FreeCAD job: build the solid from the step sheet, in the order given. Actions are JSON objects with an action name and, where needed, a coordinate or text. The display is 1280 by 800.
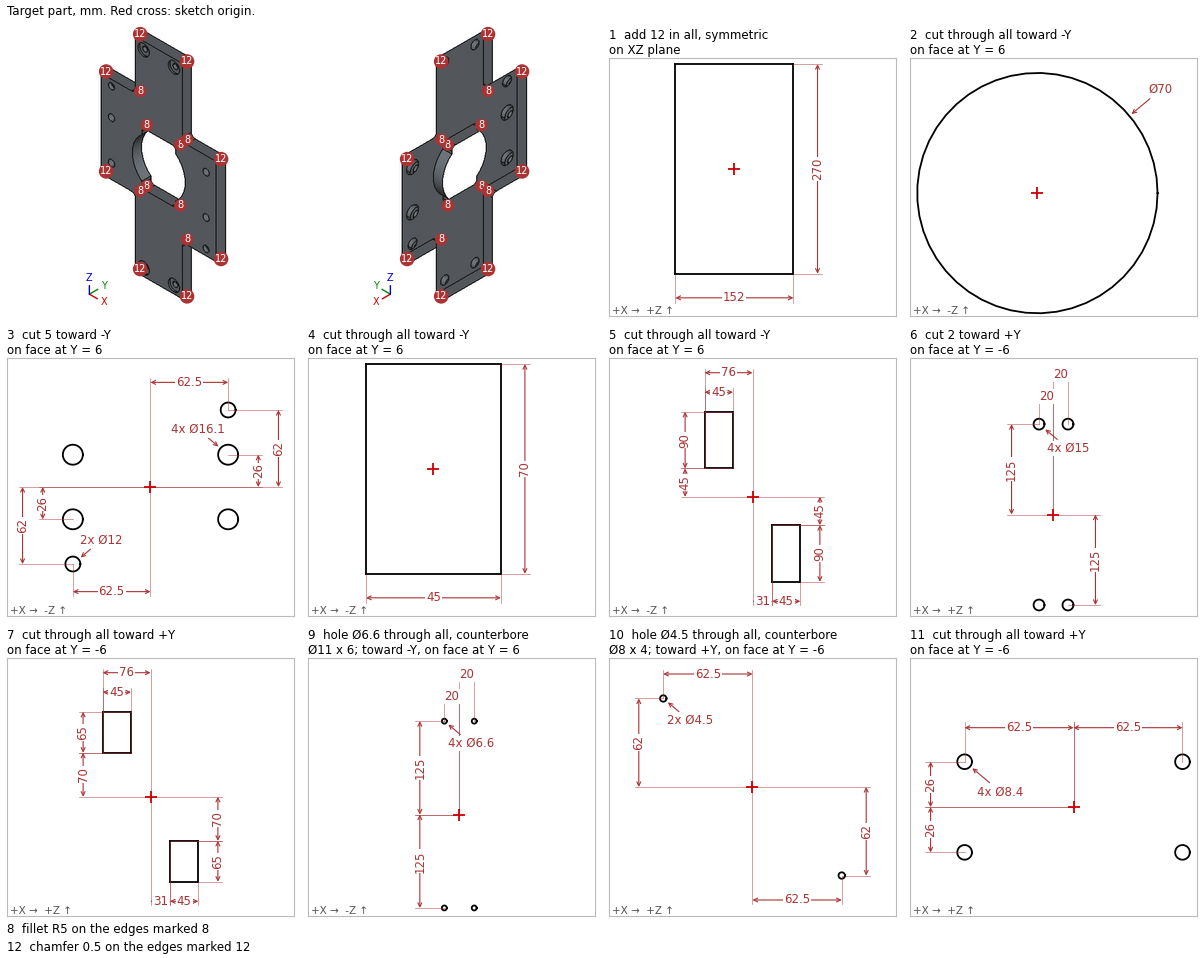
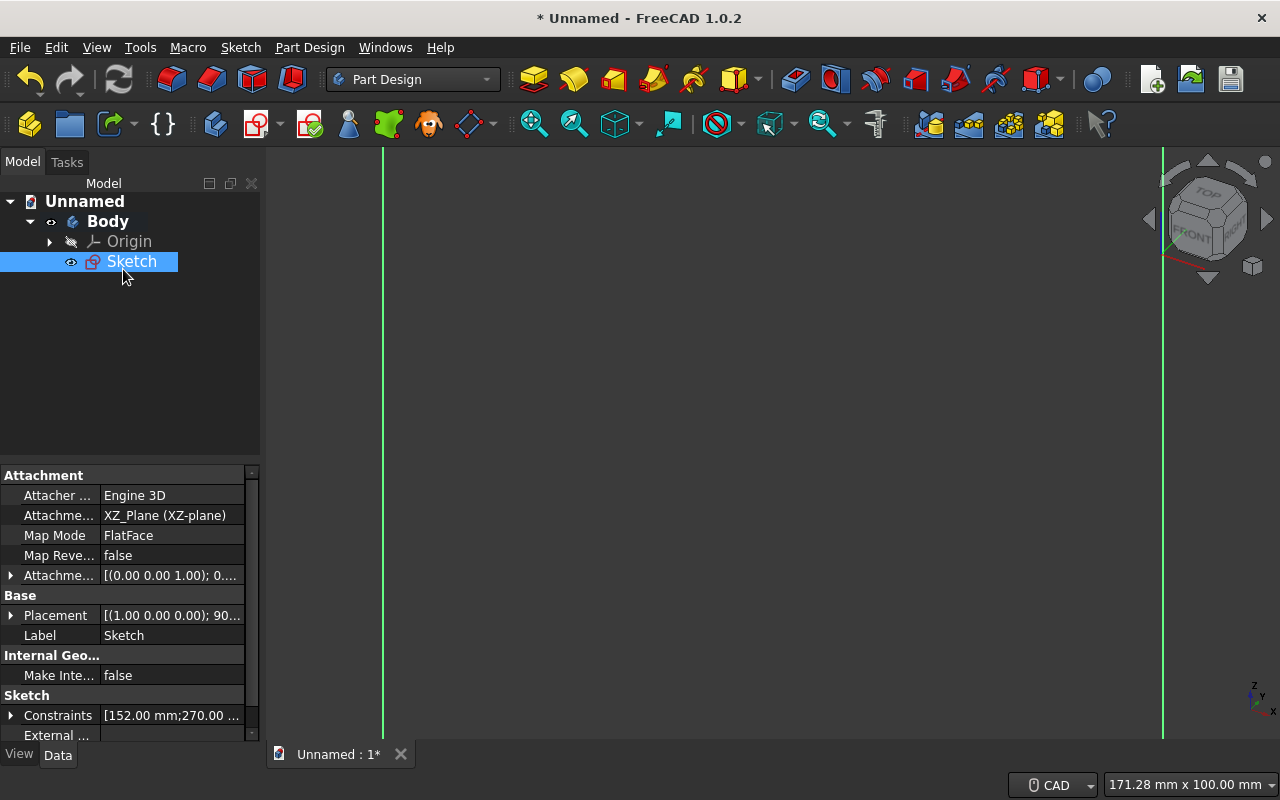
{"action": "left_click", "coordinate": [534, 80]}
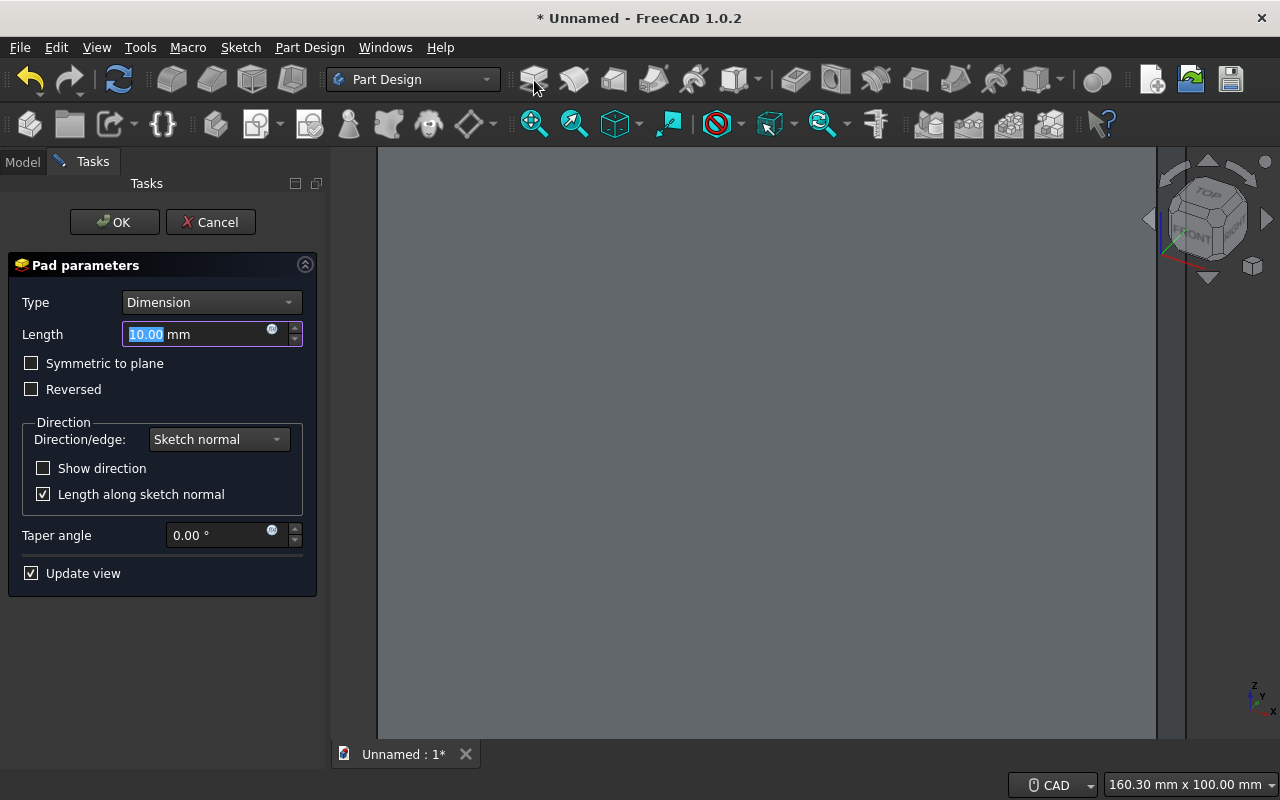
{"action": "type", "text": "12"}
{"action": "key", "text": "Tab"}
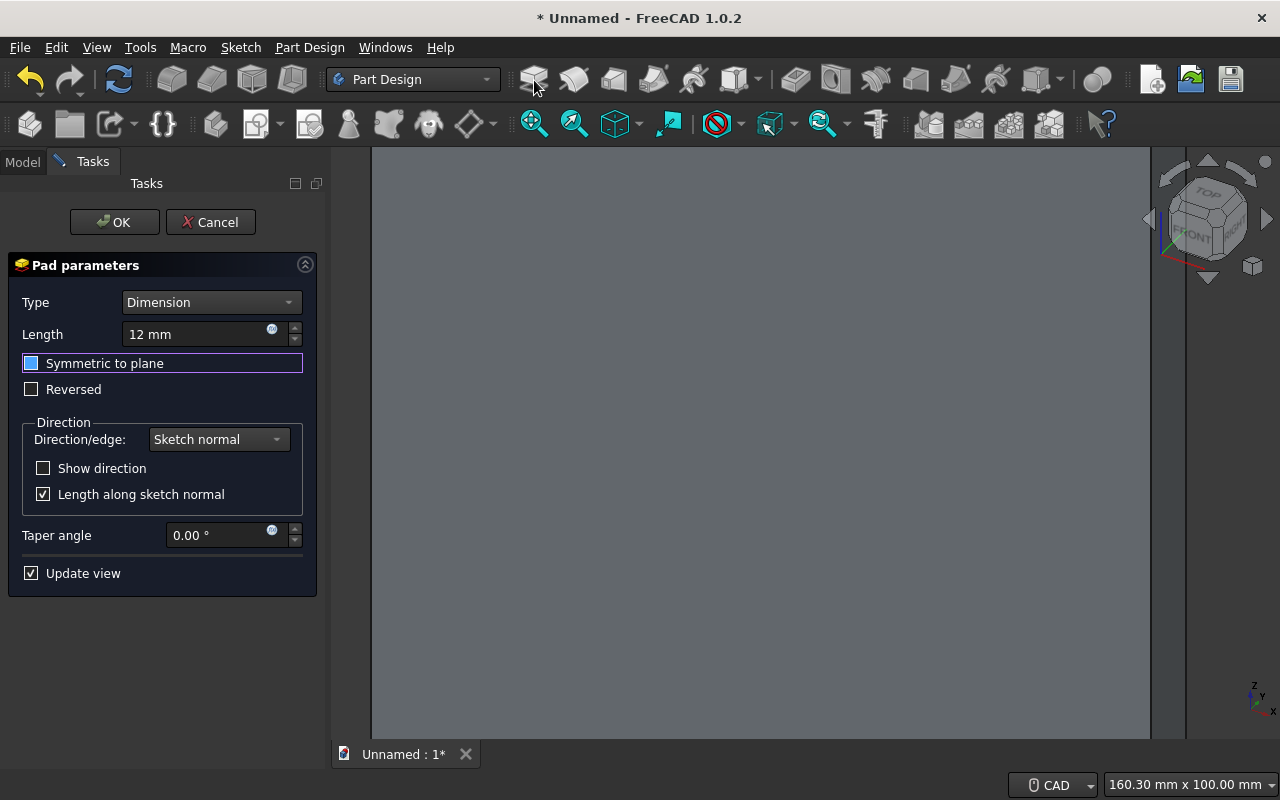
{"action": "left_click", "coordinate": [30, 363]}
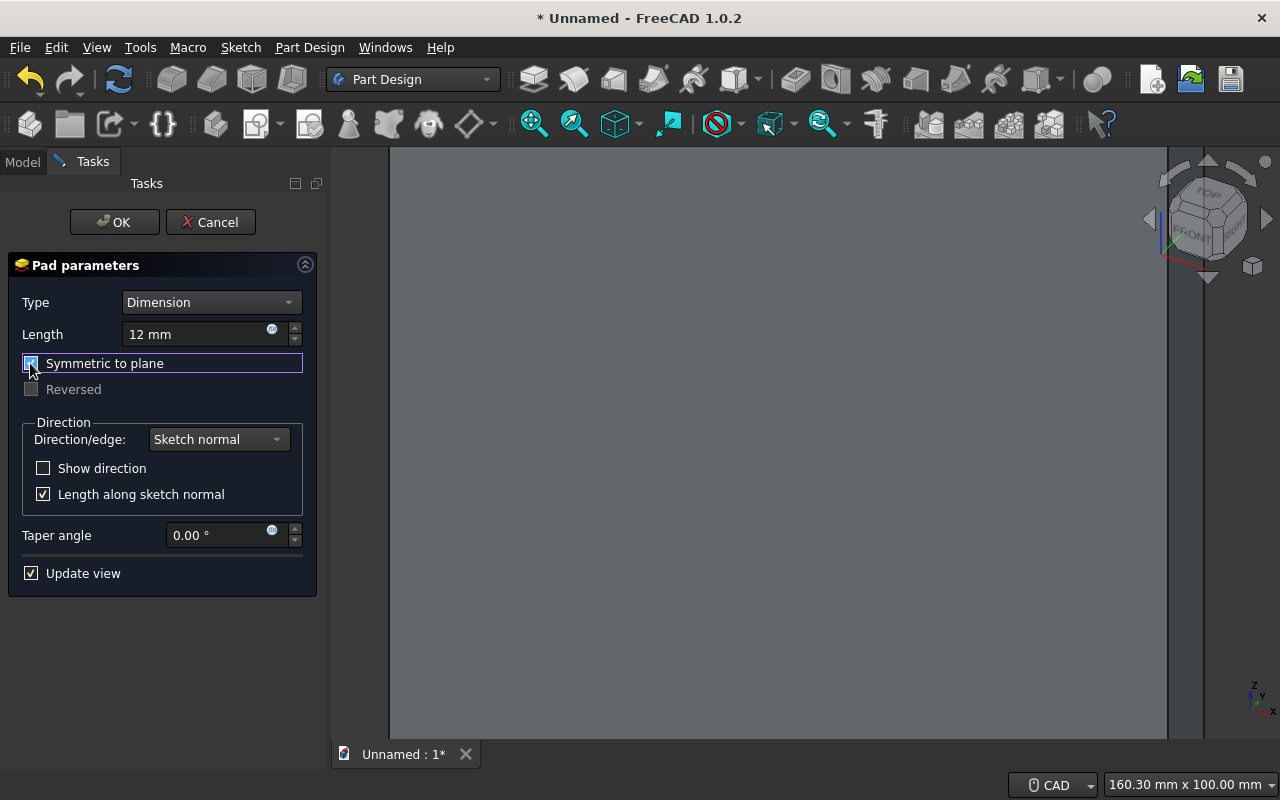
{"action": "left_click", "coordinate": [115, 222]}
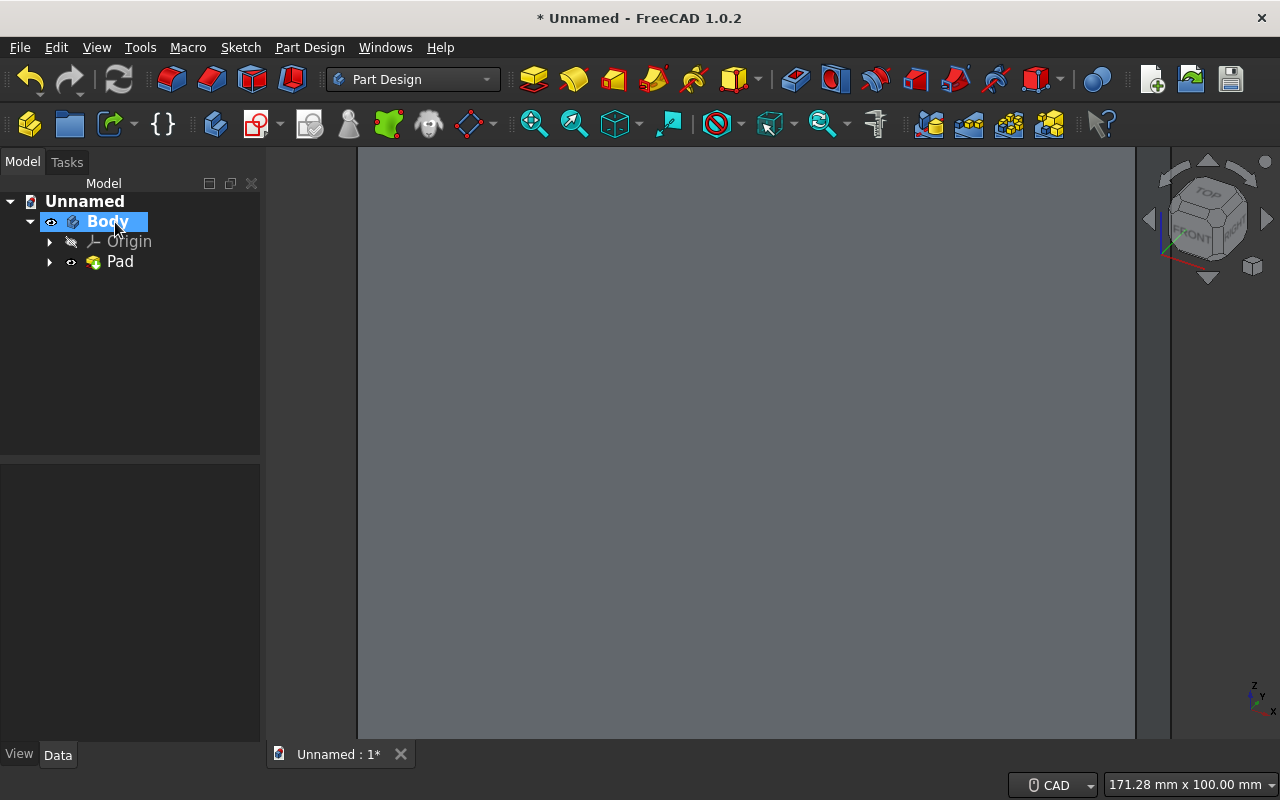
{"action": "key", "text": "v f"}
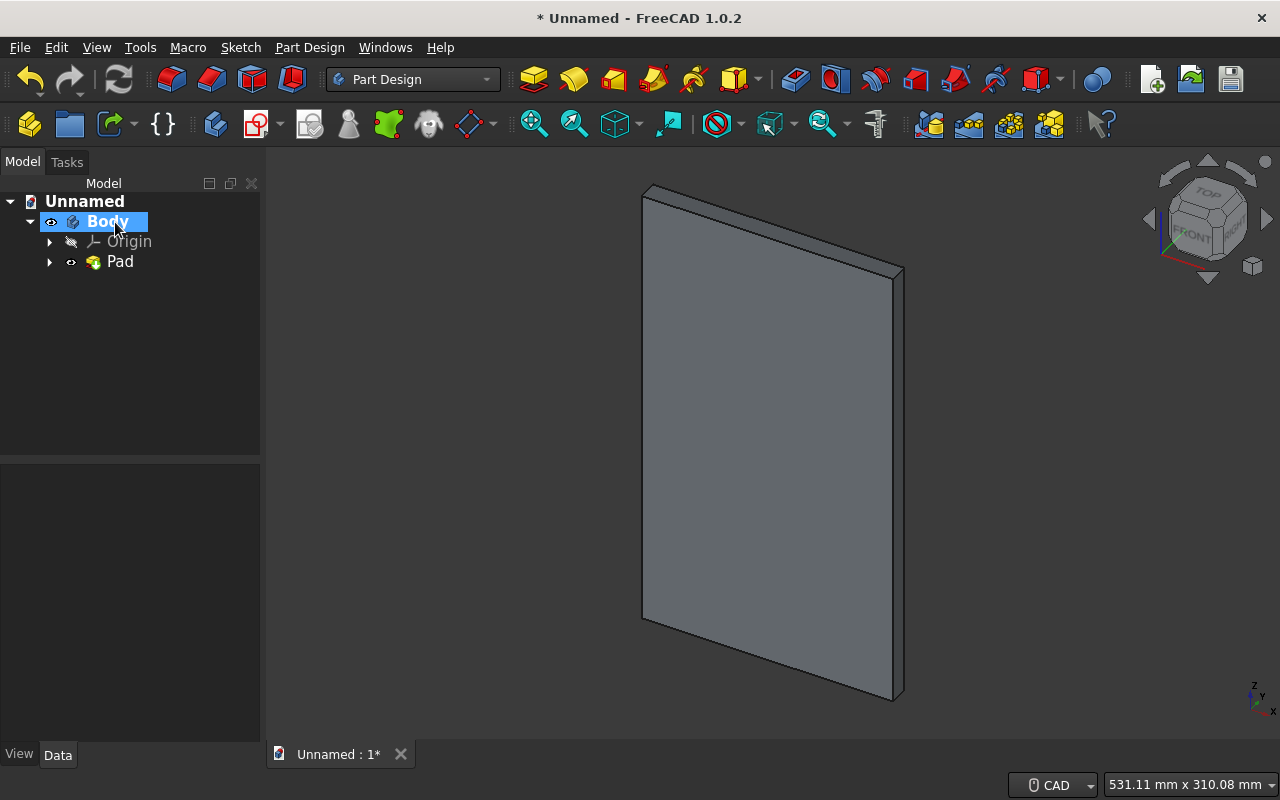
{"action": "key", "text": "4"}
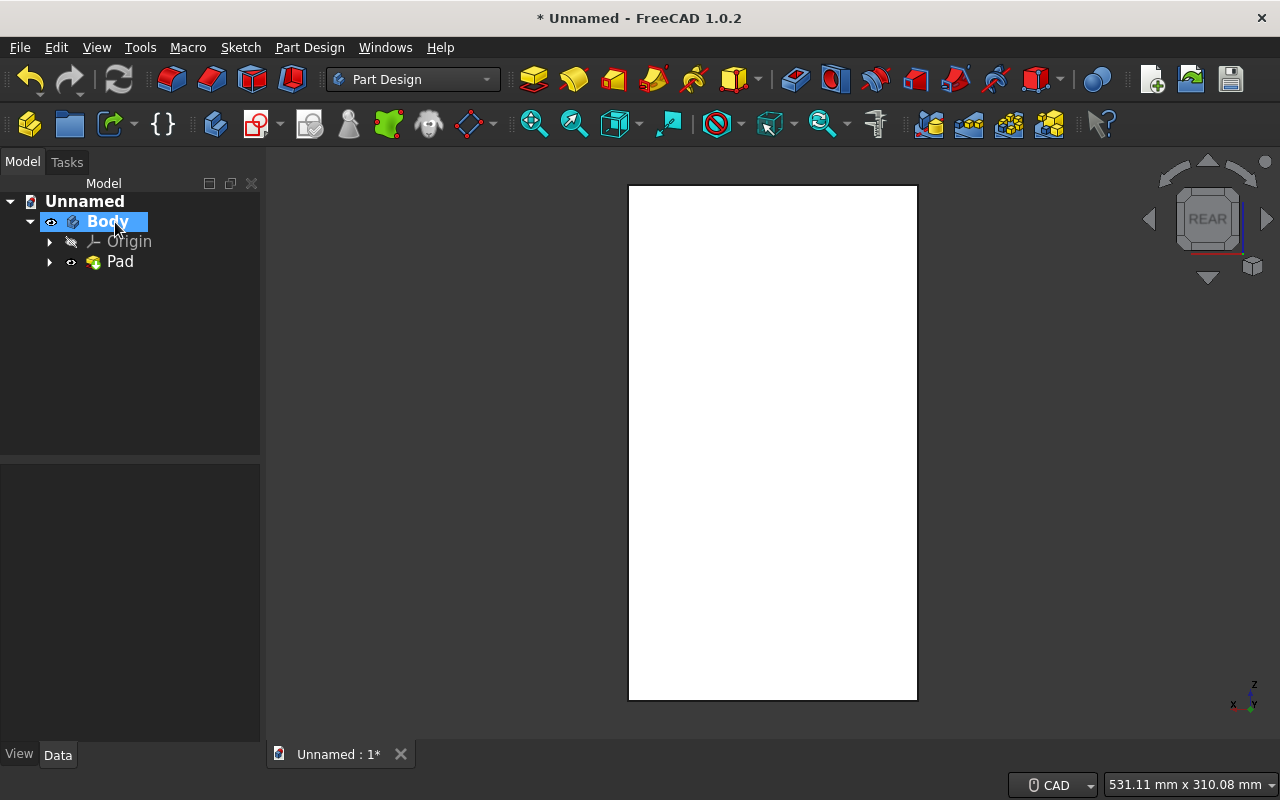
{"action": "left_click", "coordinate": [773, 368]}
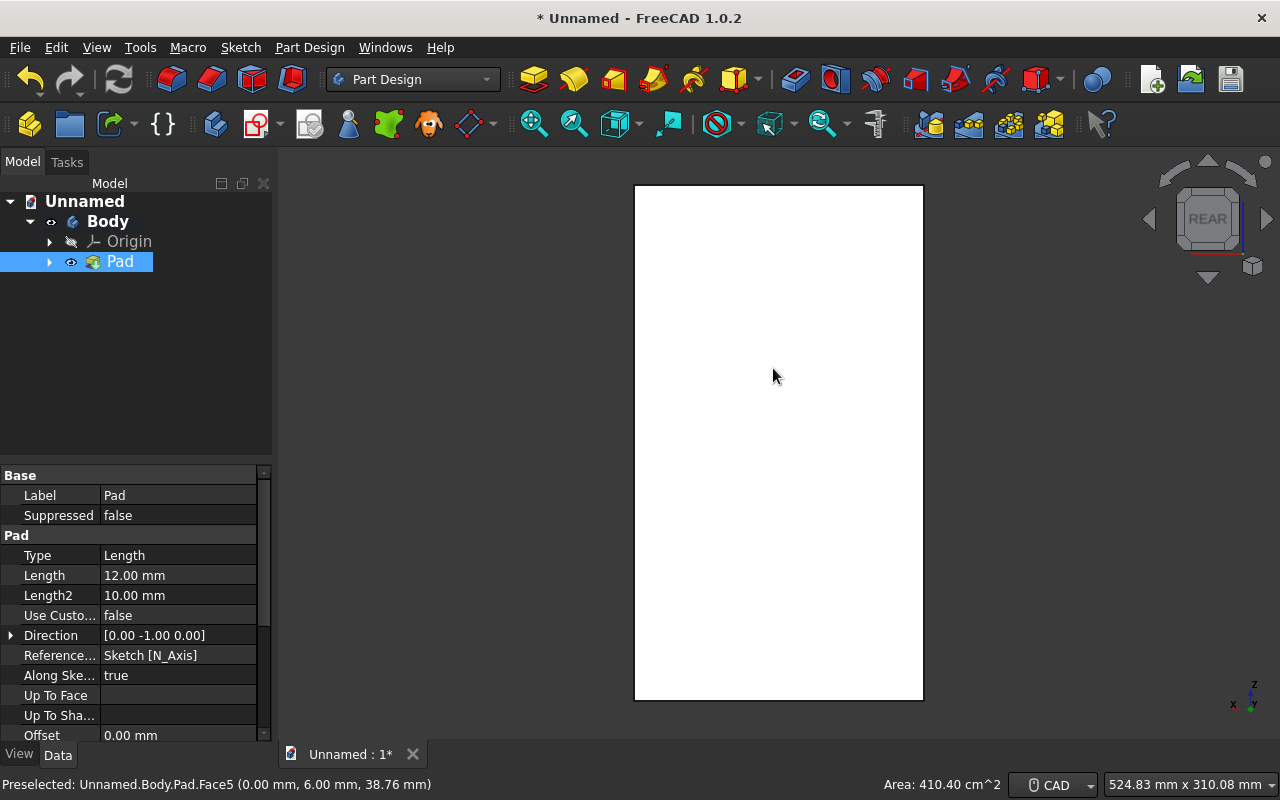
{"action": "left_click", "coordinate": [256, 124]}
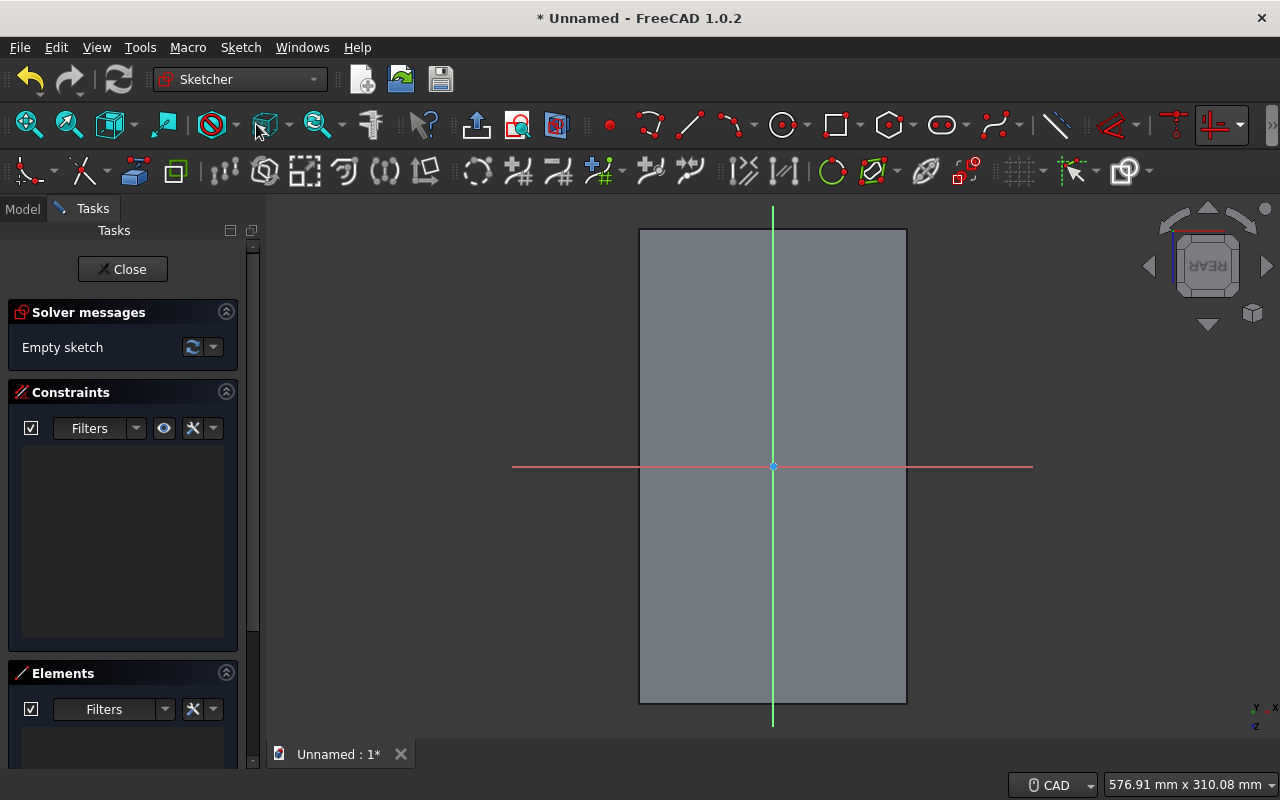
{"action": "scroll", "coordinate": [813, 467], "scroll_direction": "up", "scroll_amount": 5}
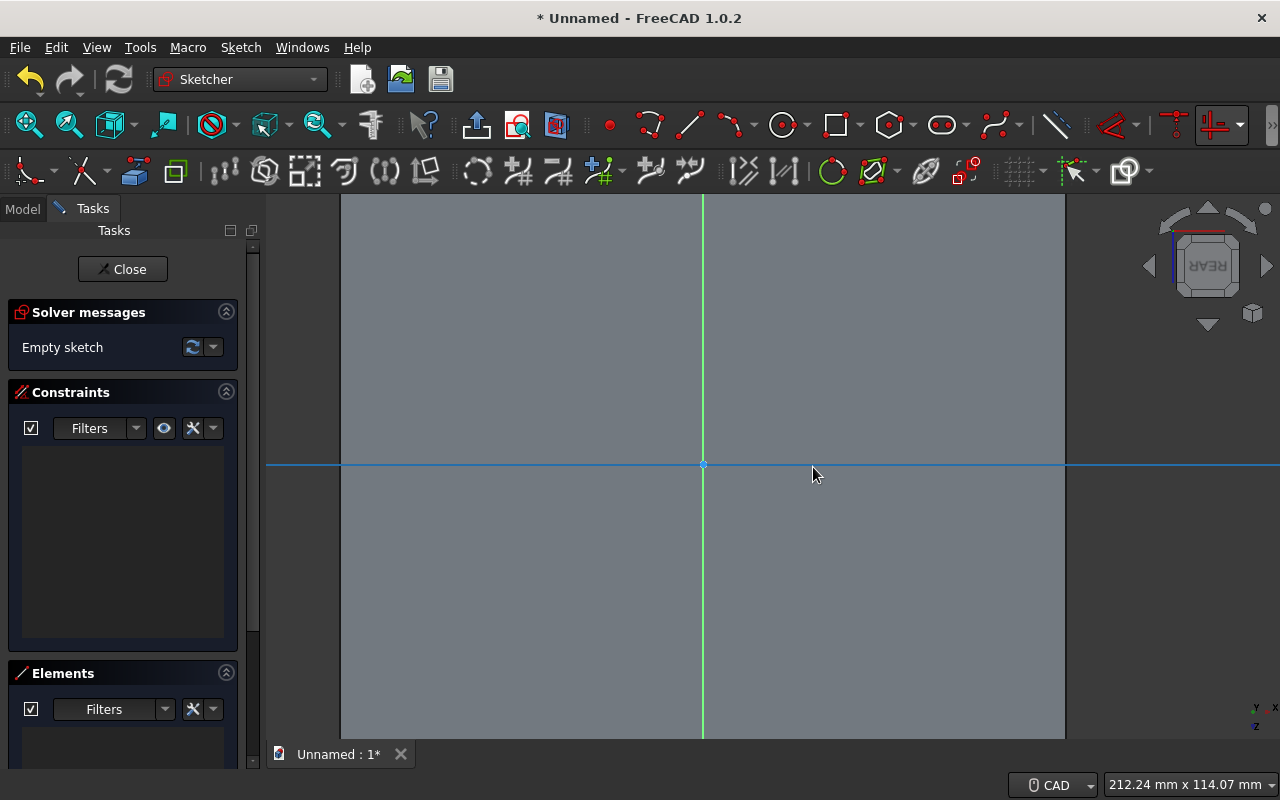
{"action": "key", "text": "g c"}